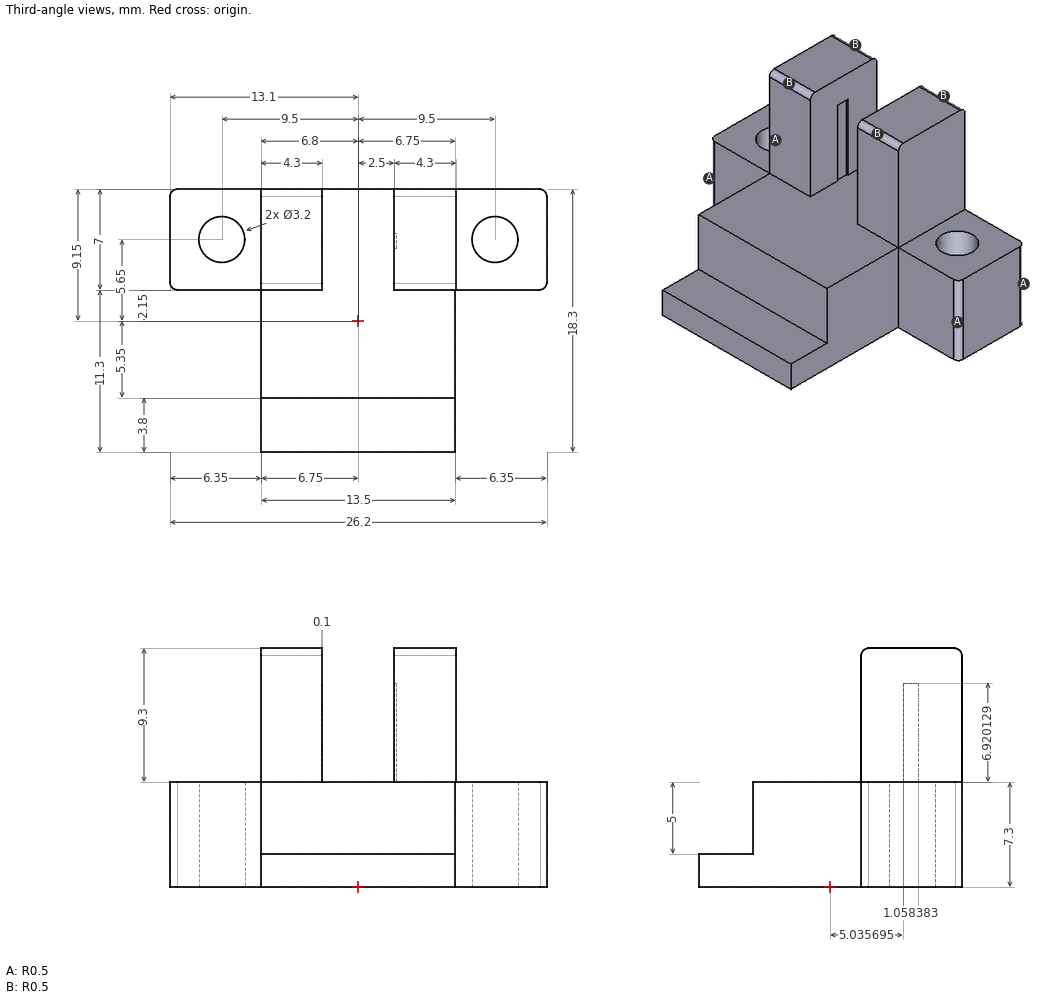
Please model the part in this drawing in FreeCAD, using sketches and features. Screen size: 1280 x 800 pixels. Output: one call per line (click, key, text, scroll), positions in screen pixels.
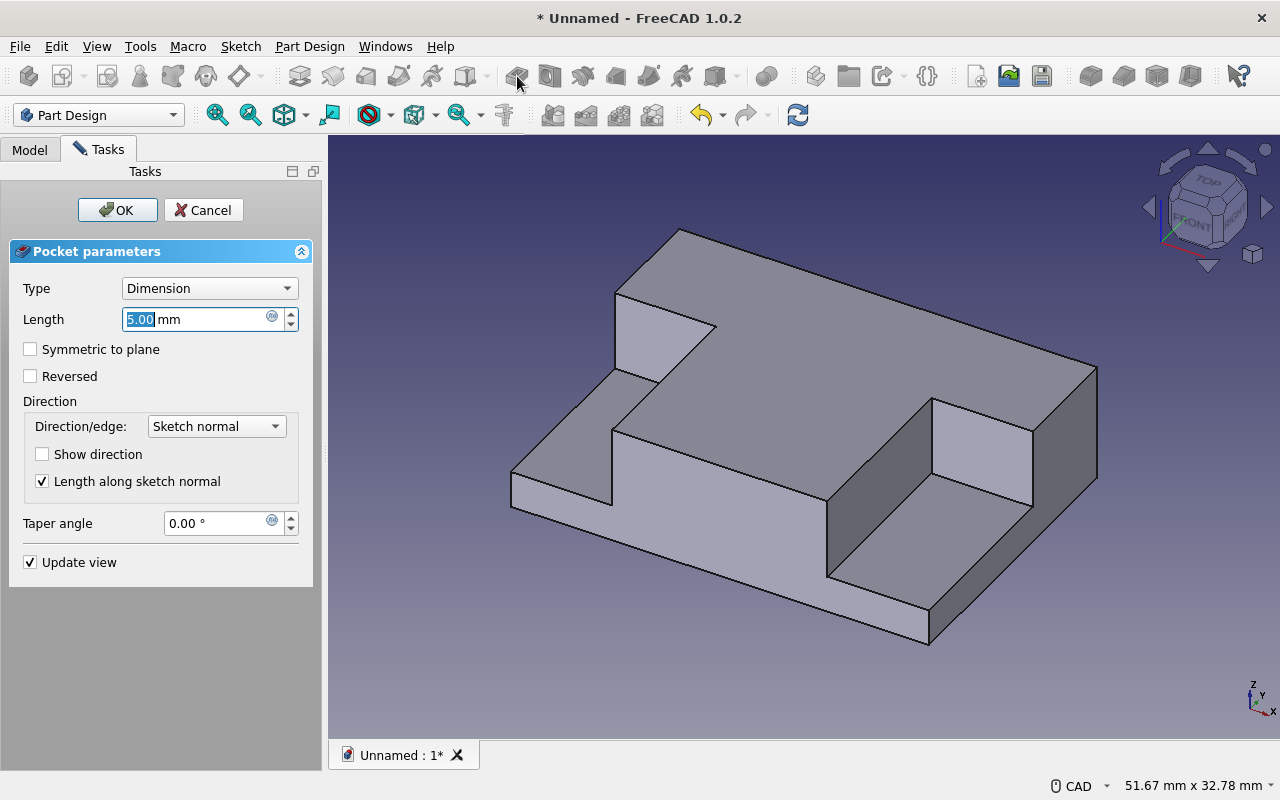
click(210, 288)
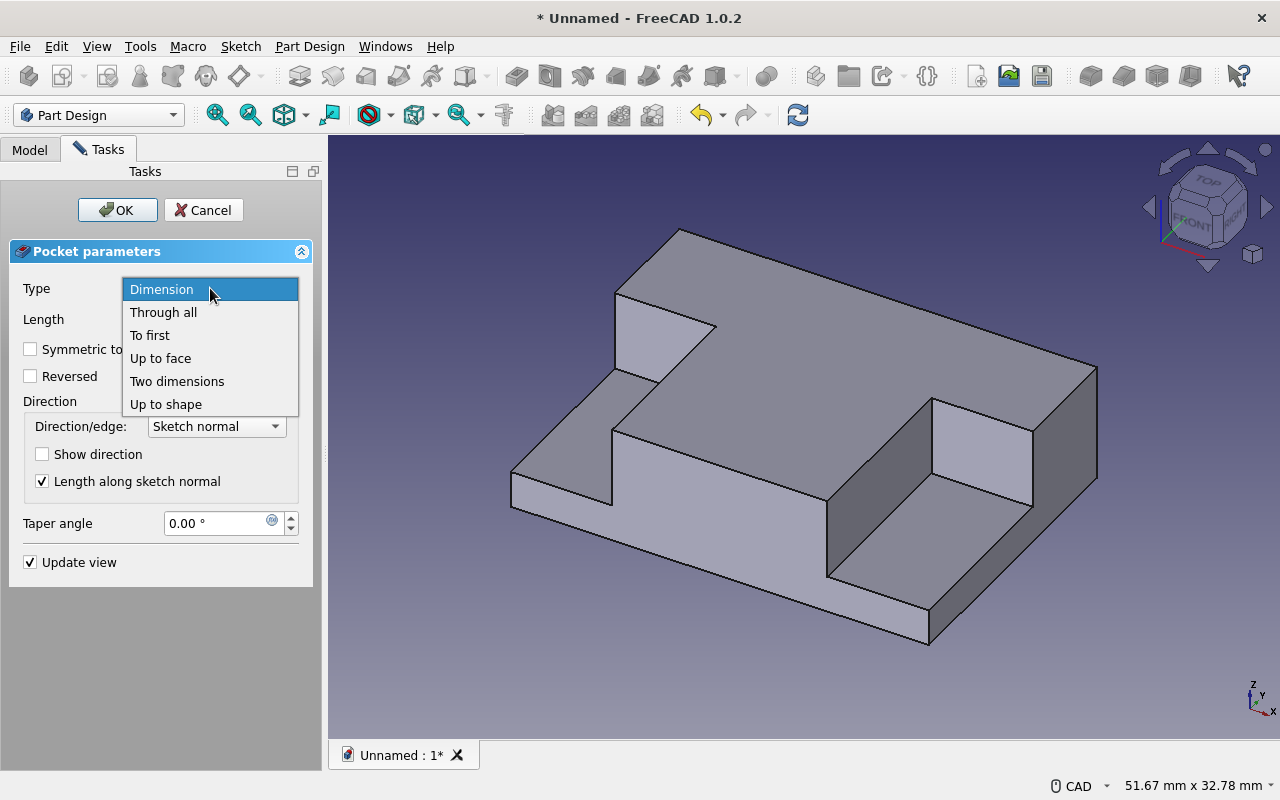
click(208, 312)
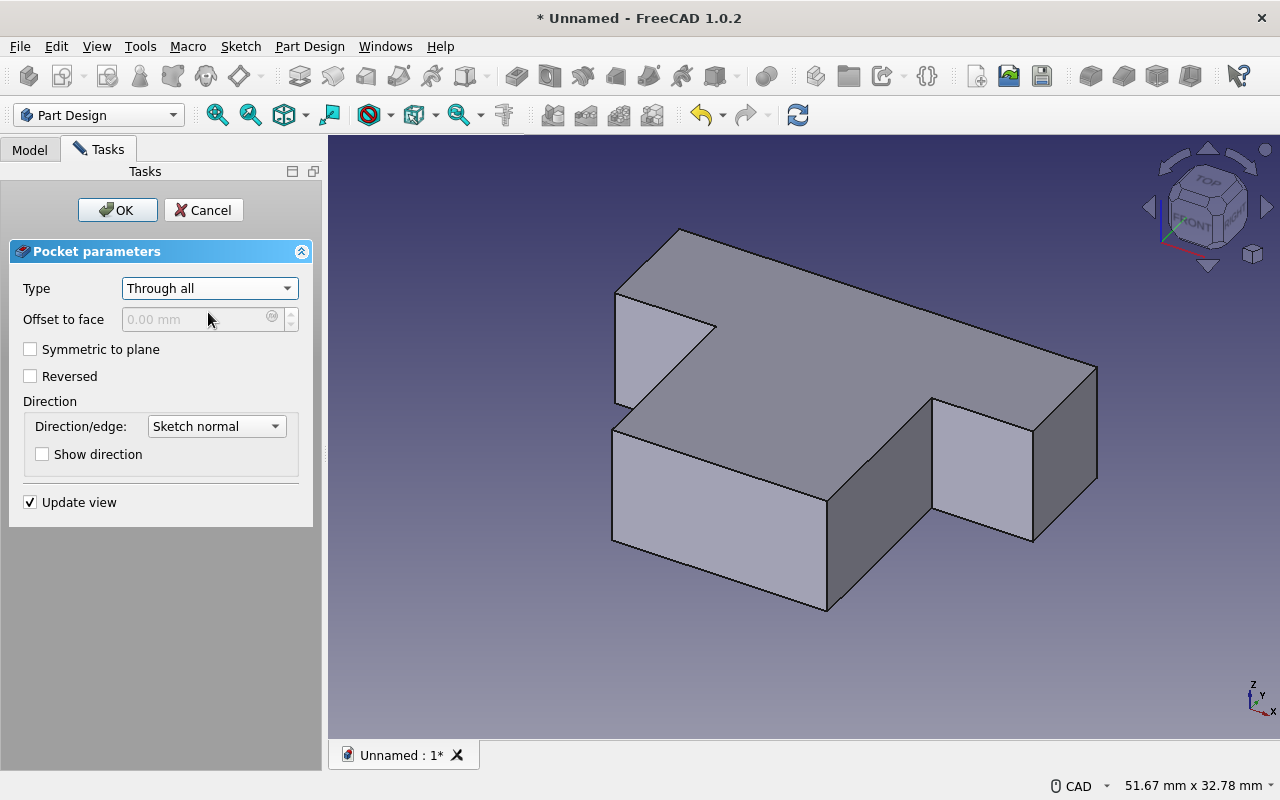
click(118, 210)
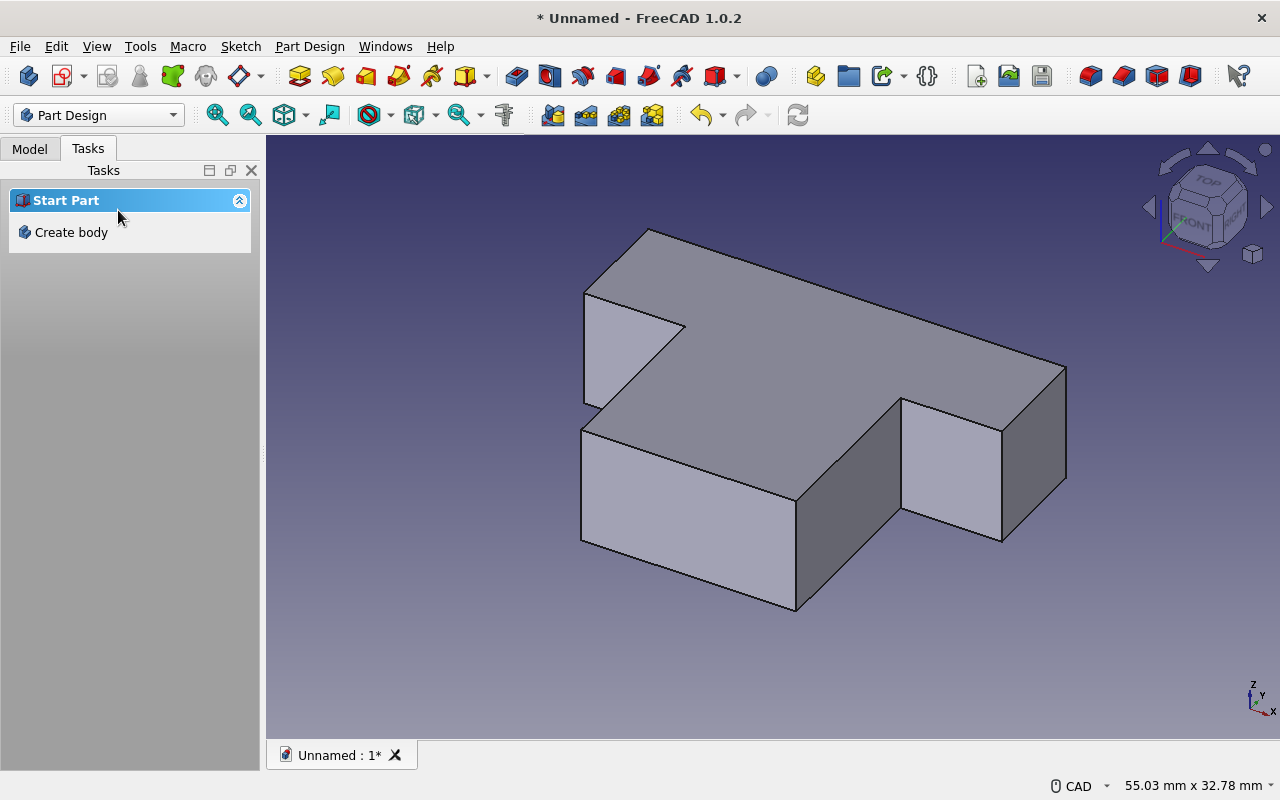
click(773, 381)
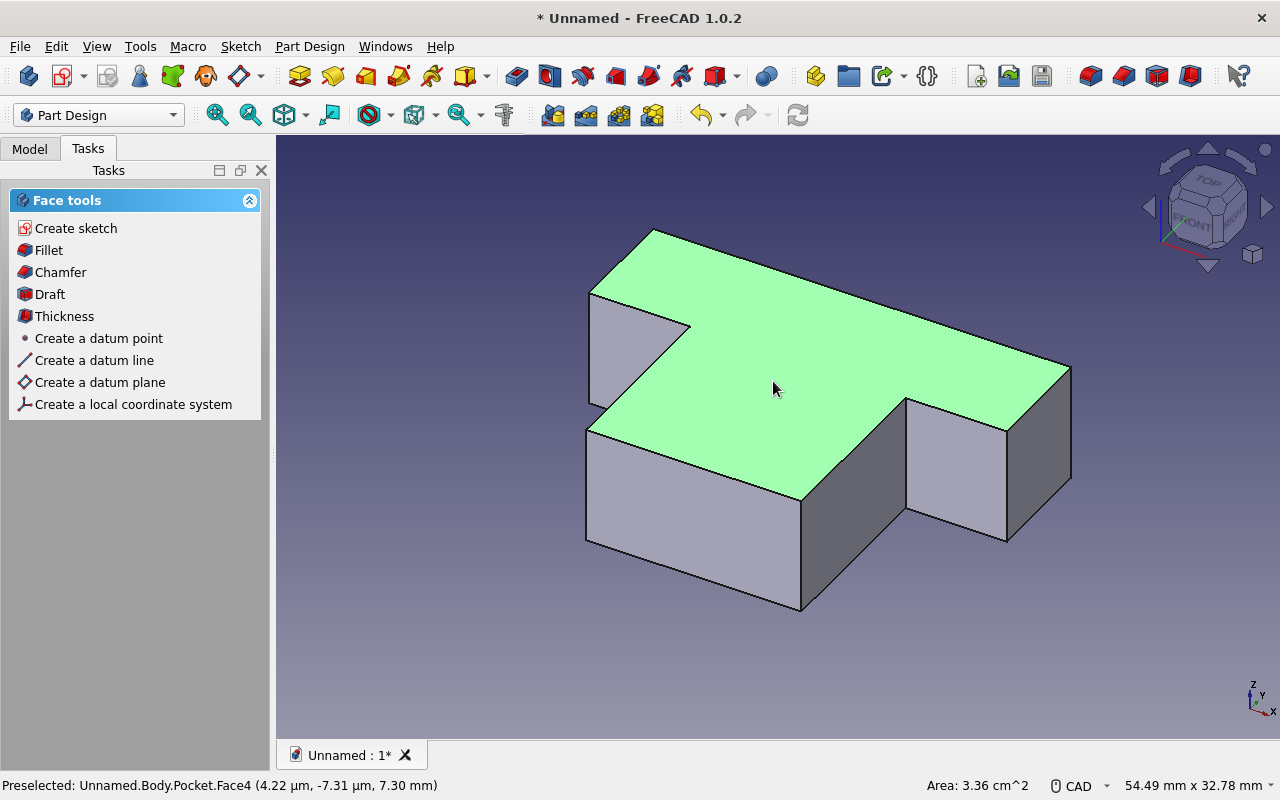
click(62, 76)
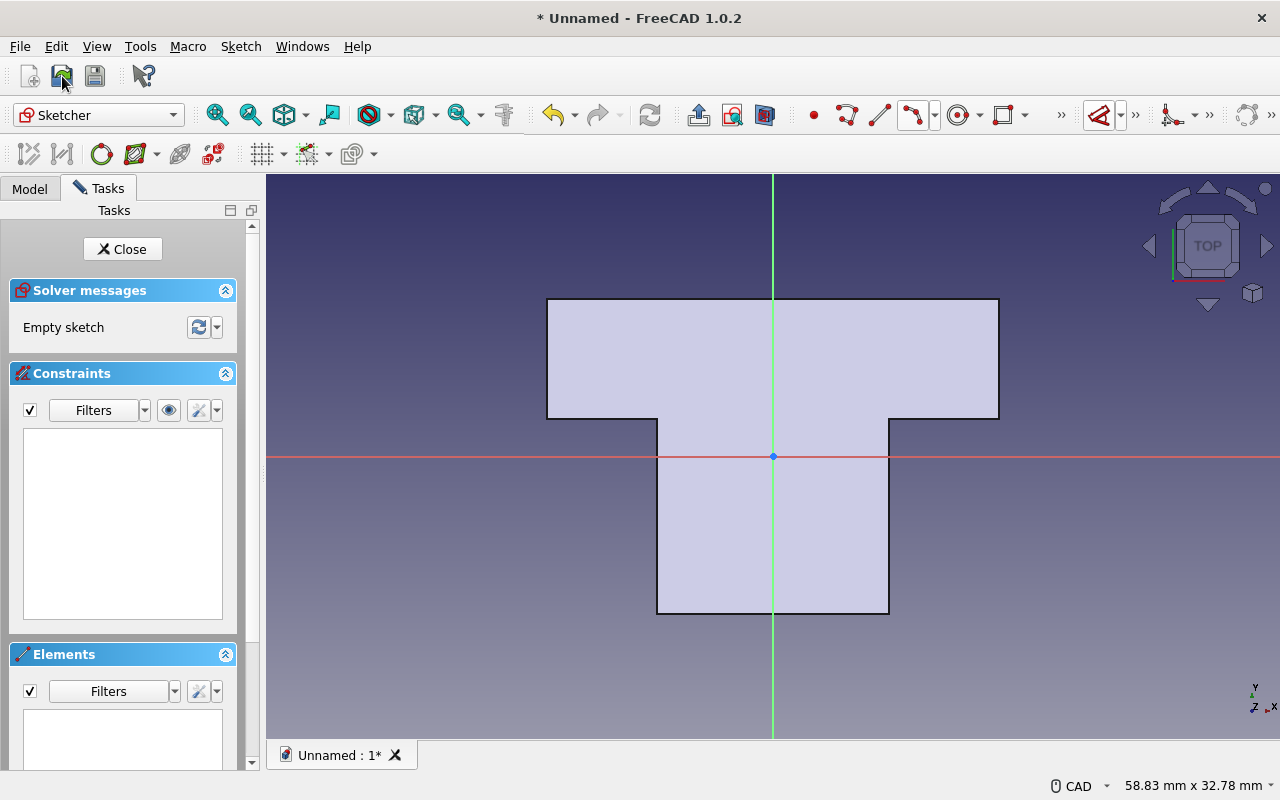
scroll(829, 313, up, 4)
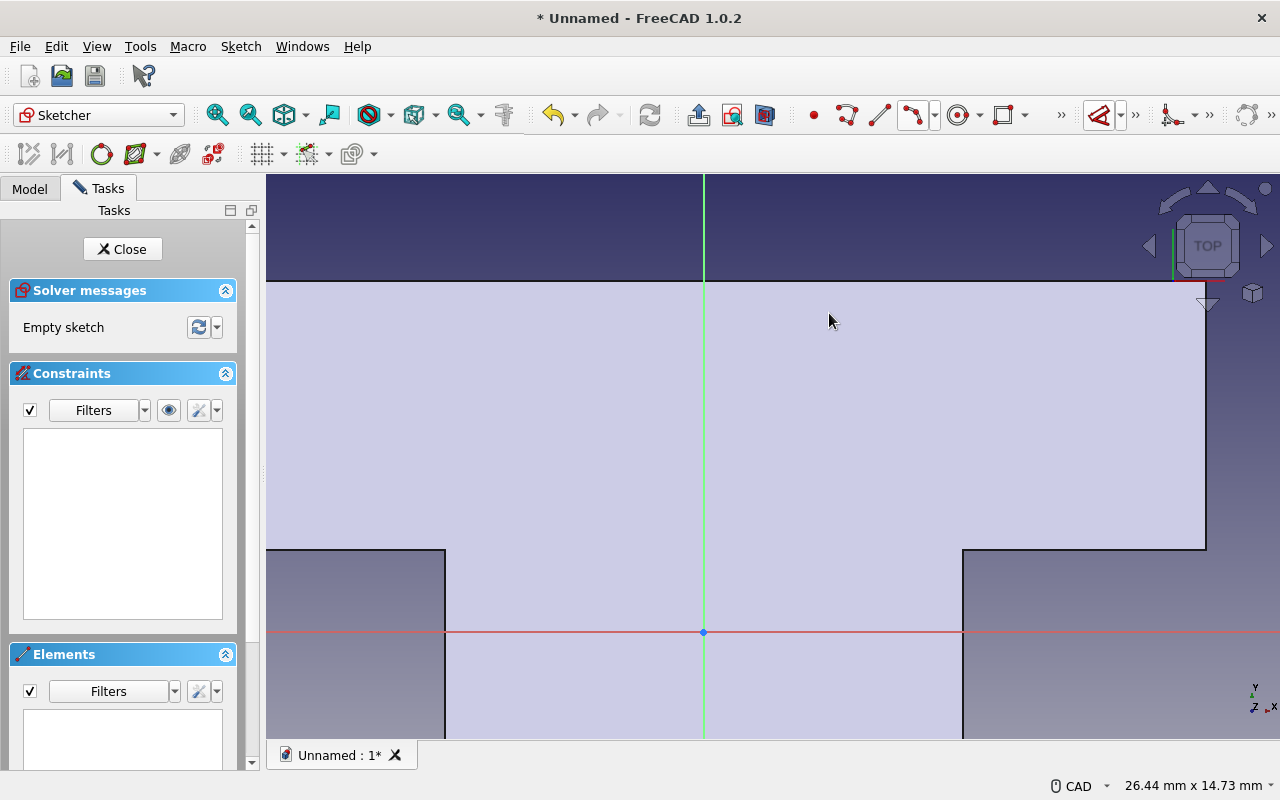
key(g)
key(r)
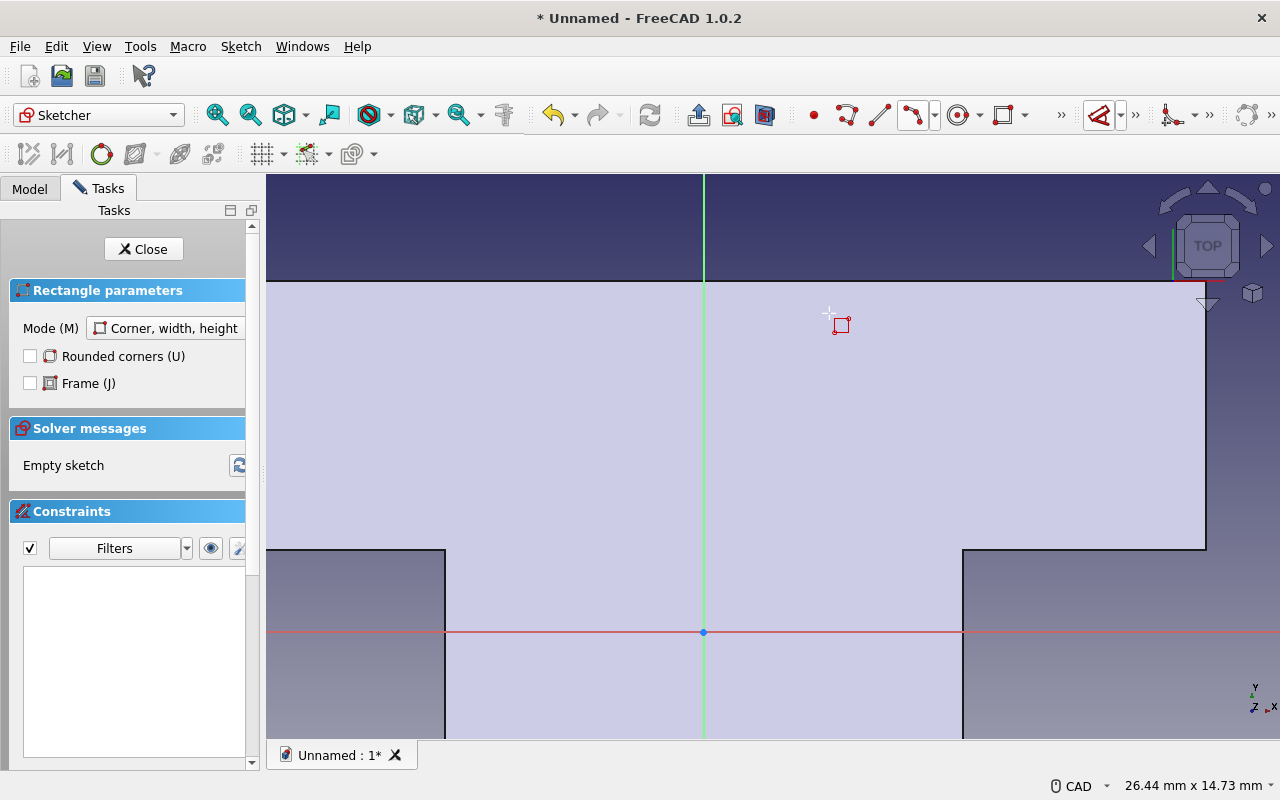
click(443, 281)
click(608, 550)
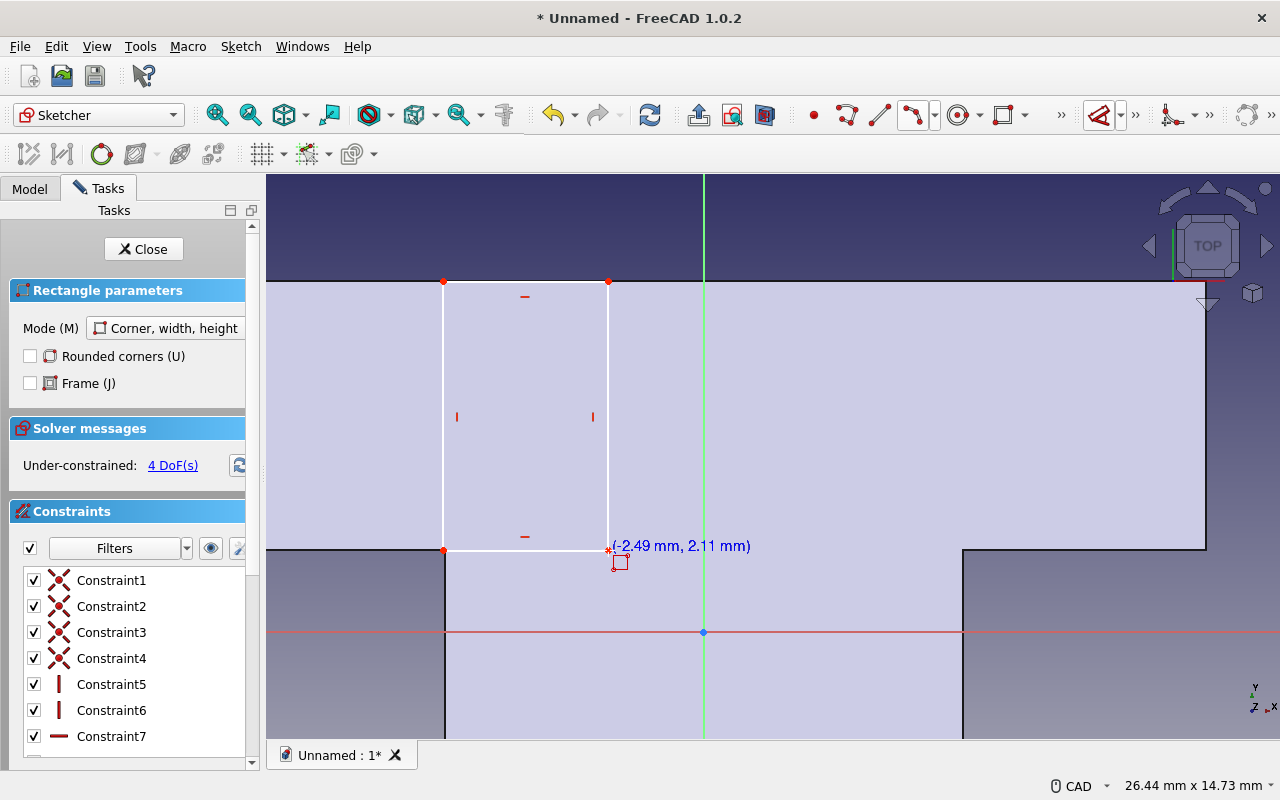
click(800, 281)
click(965, 550)
key(Escape)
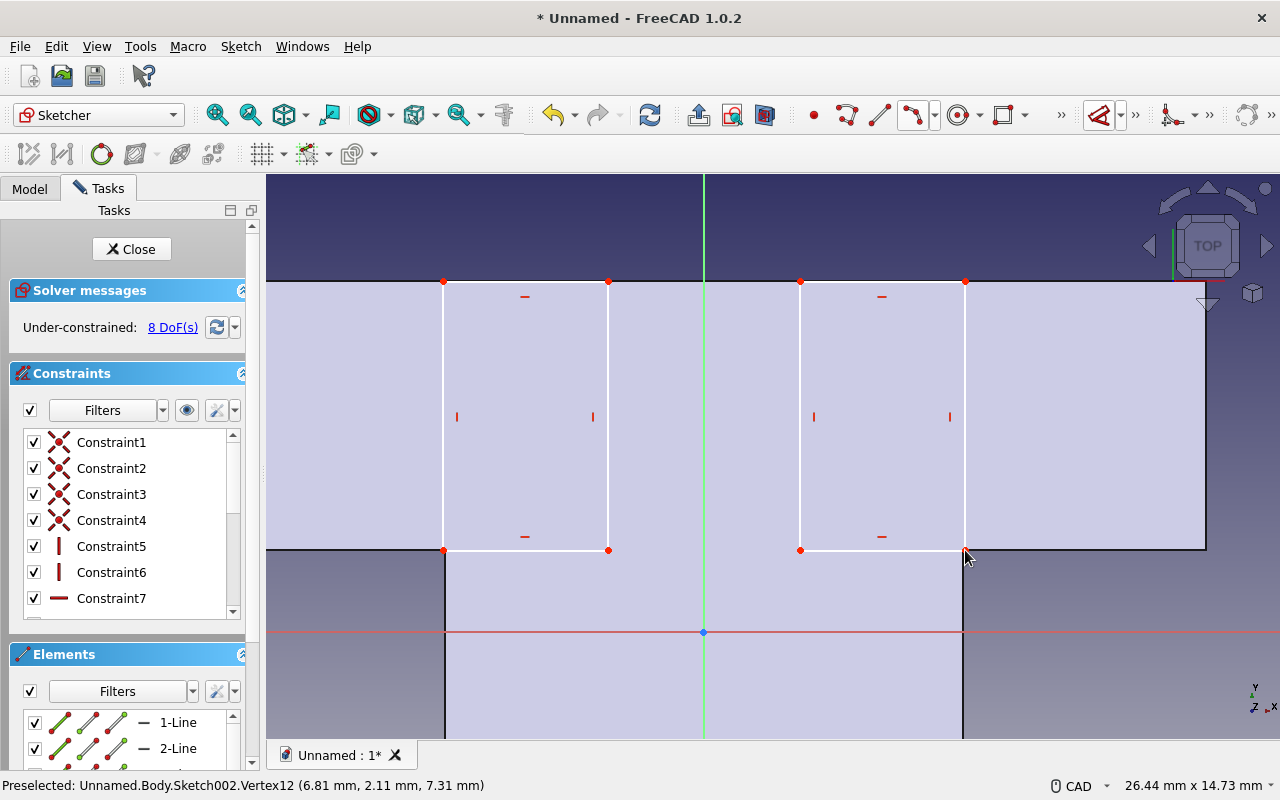
click(443, 363)